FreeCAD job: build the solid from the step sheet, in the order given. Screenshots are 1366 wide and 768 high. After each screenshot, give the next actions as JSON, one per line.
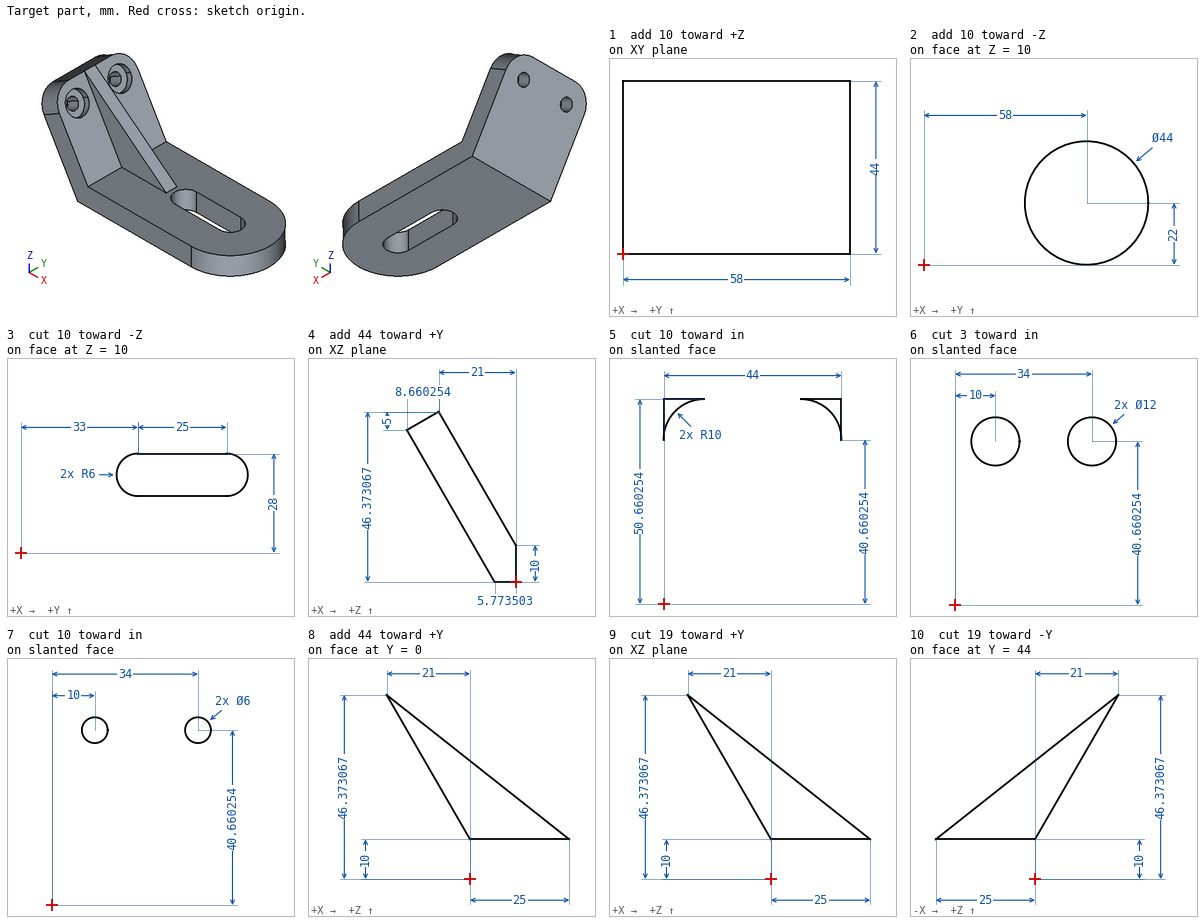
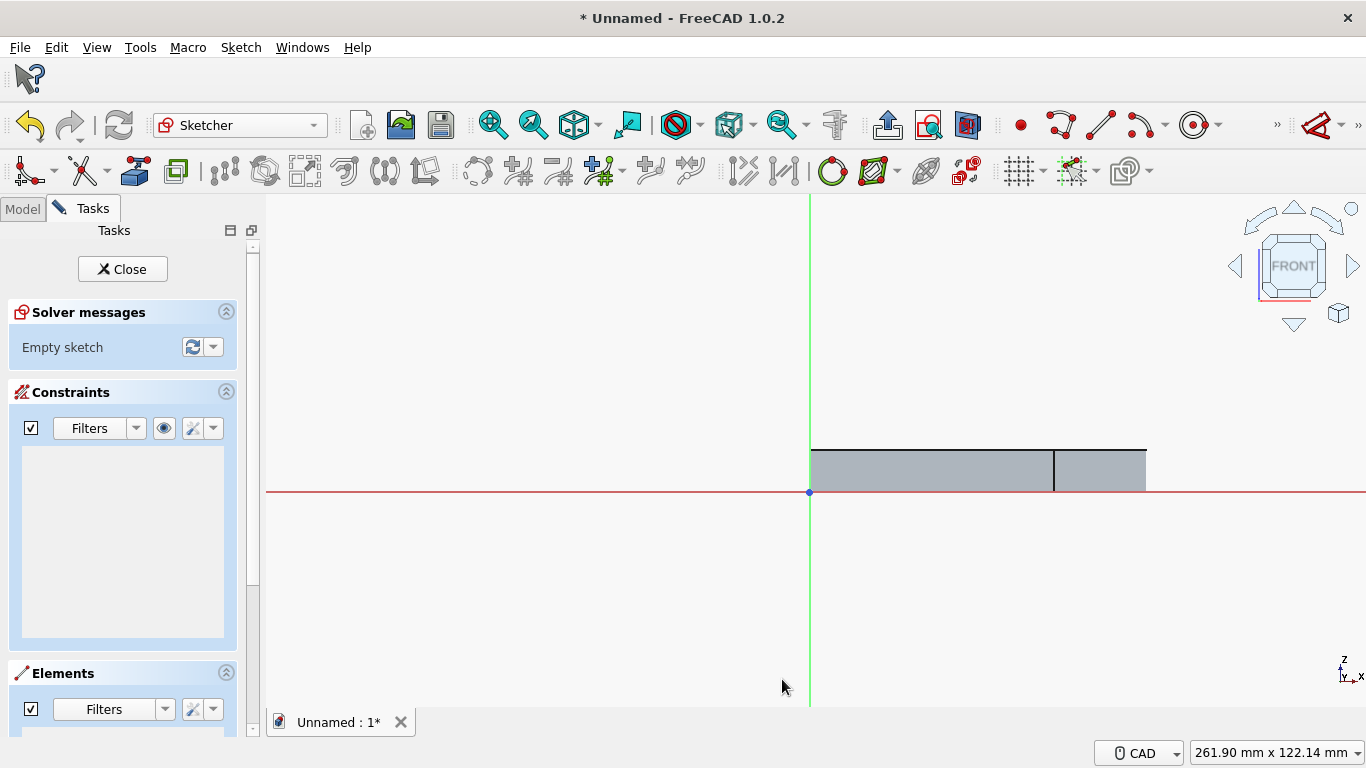
{"action": "scroll", "coordinate": [748, 327], "scroll_direction": "up", "scroll_amount": 3}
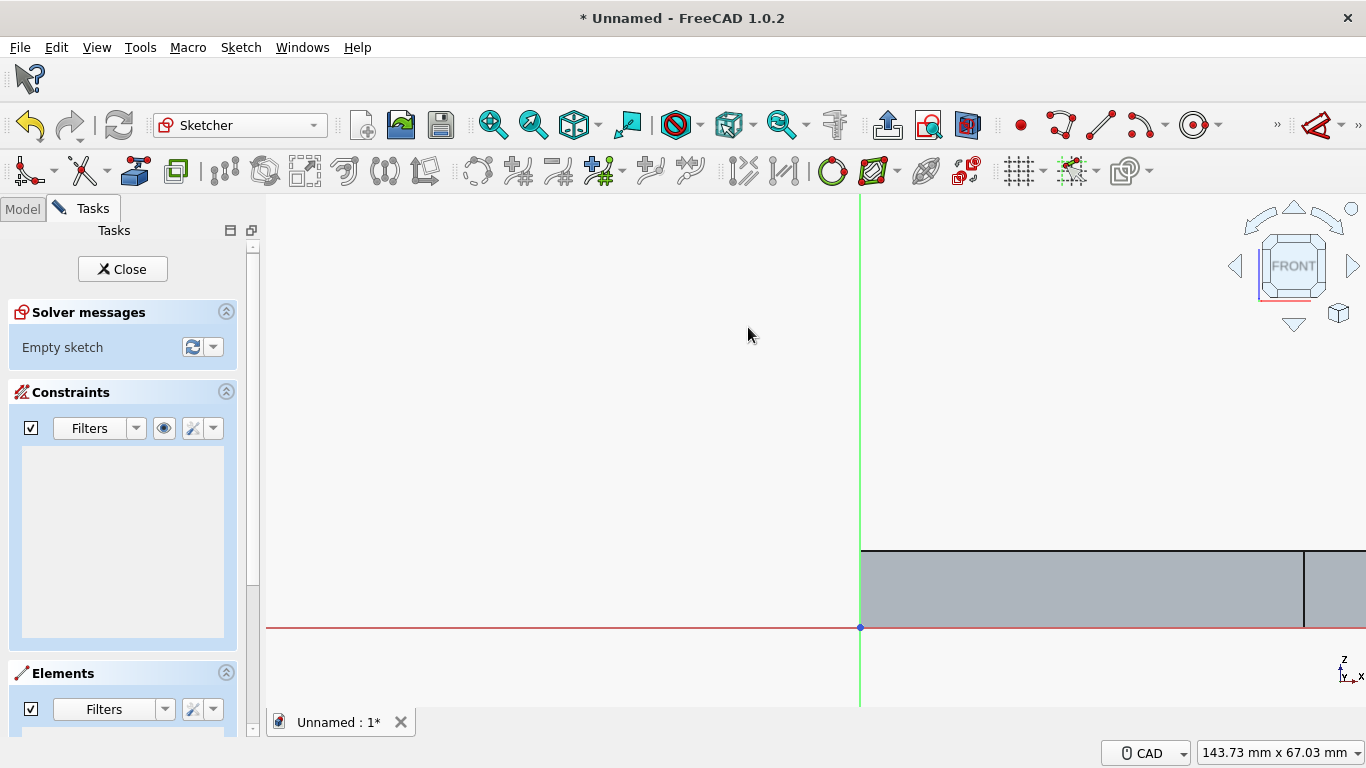
{"action": "left_click", "coordinate": [1062, 126]}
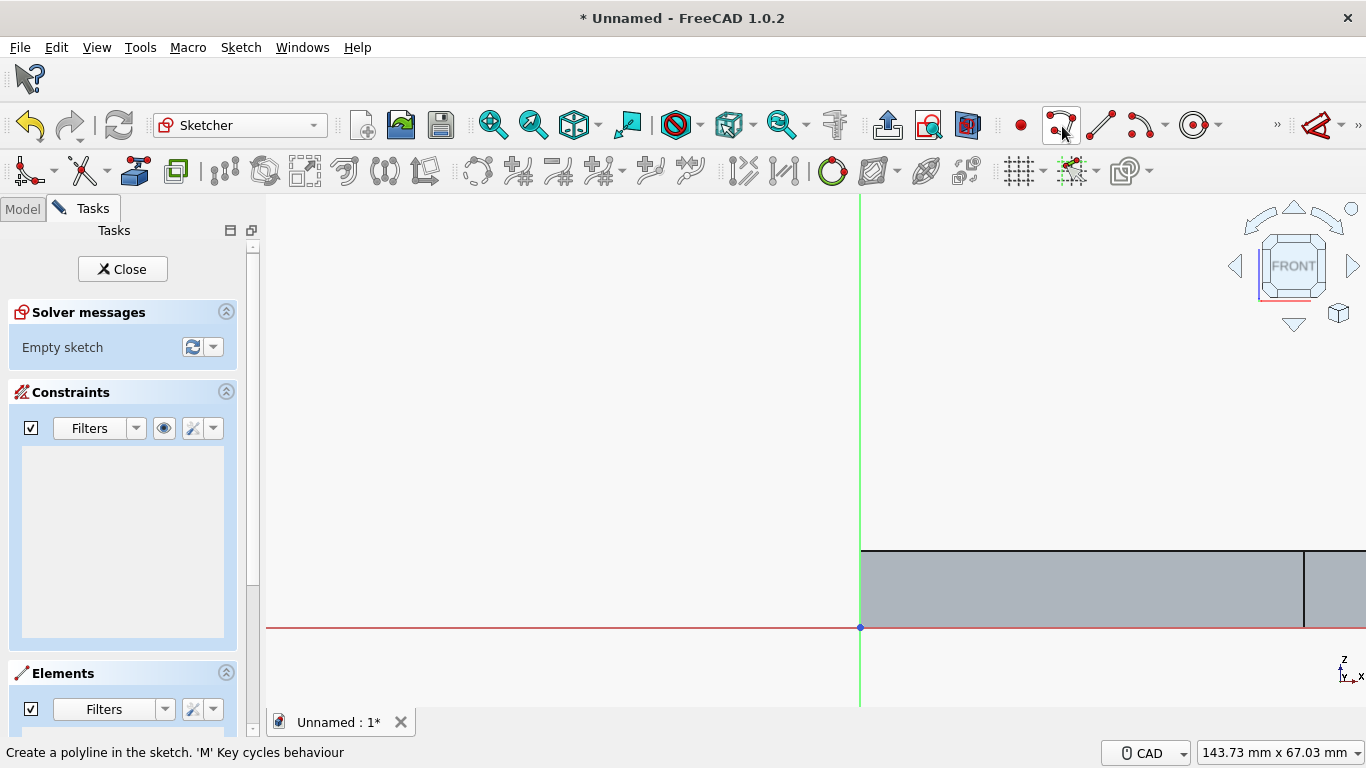
{"action": "left_click", "coordinate": [860, 628]}
{"action": "left_click", "coordinate": [851, 551]}
{"action": "left_click", "coordinate": [700, 273]}
{"action": "left_click", "coordinate": [633, 311]}
{"action": "left_click", "coordinate": [816, 619]}
{"action": "left_click", "coordinate": [860, 628]}
{"action": "key", "text": "Escape"}
{"action": "key", "text": "Escape"}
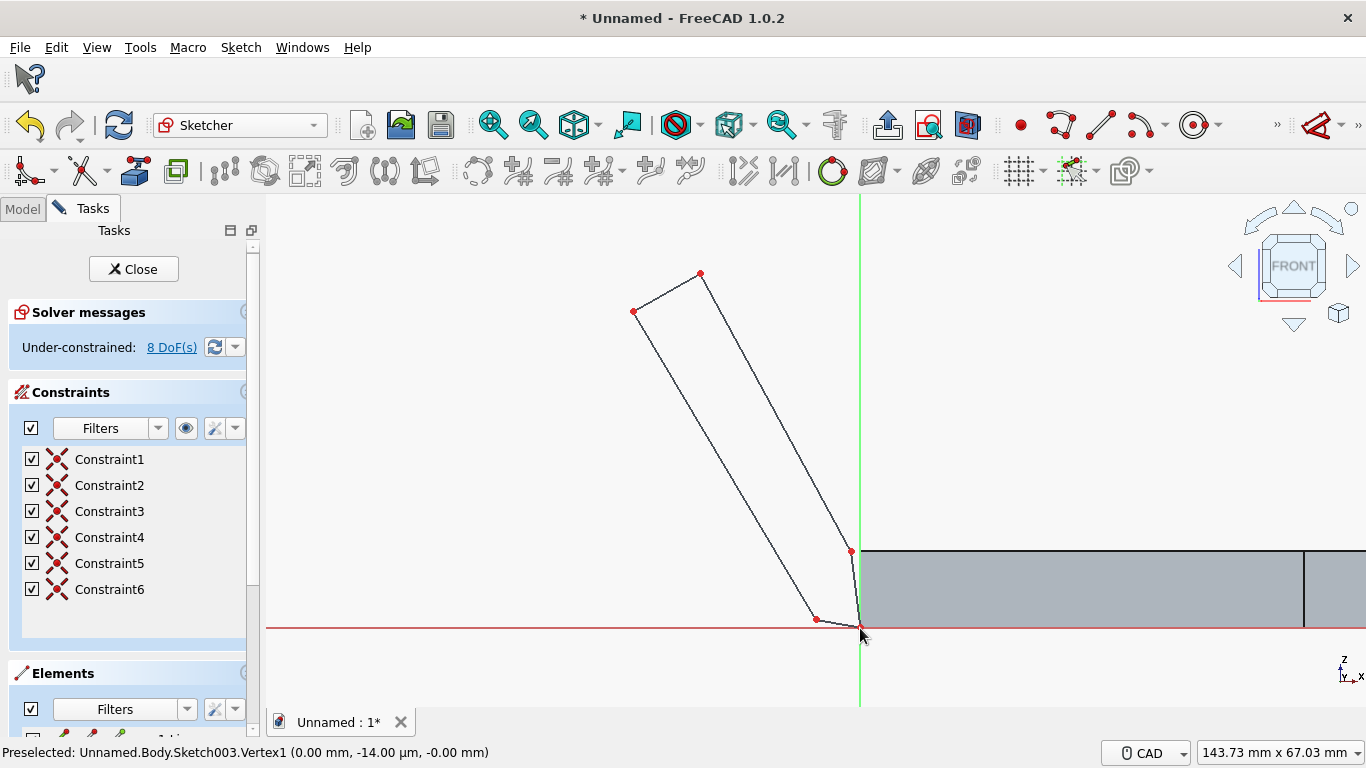
{"action": "left_click", "coordinate": [858, 605]}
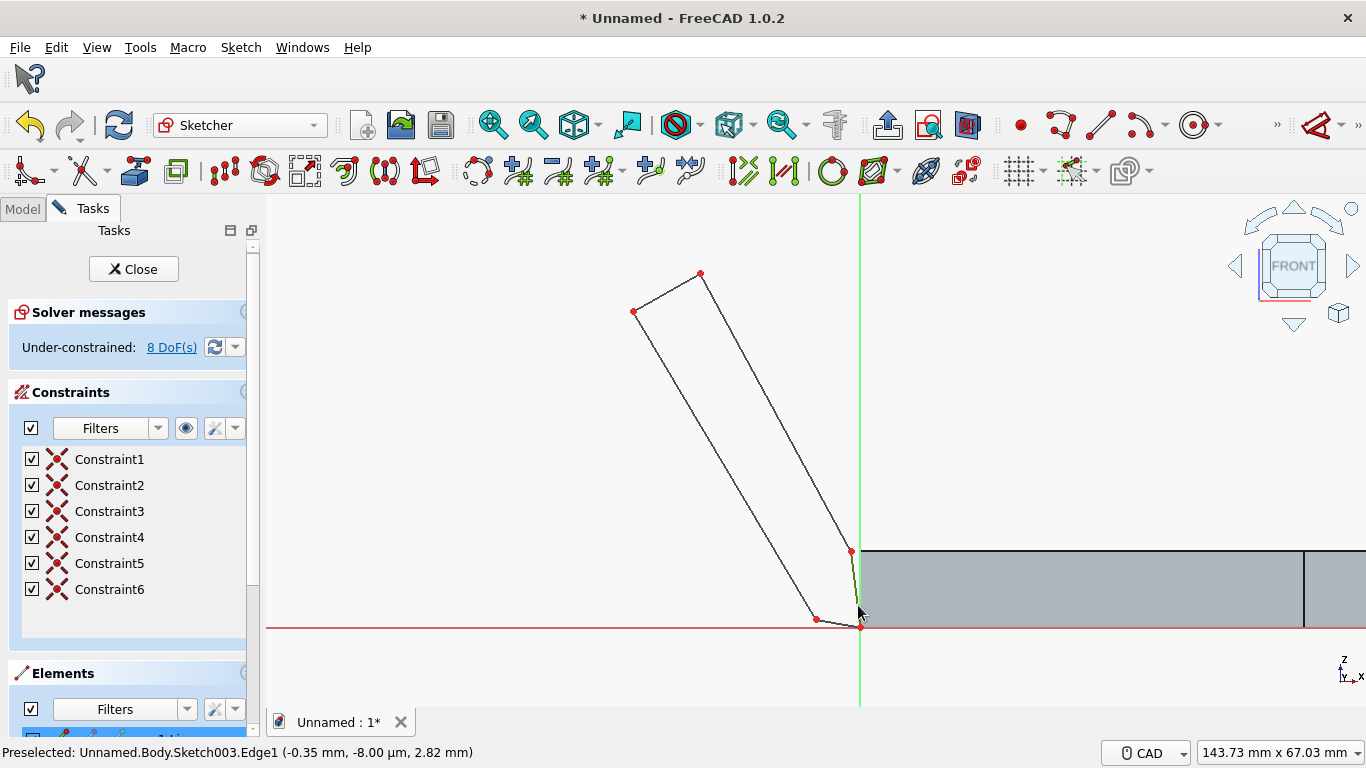
{"action": "key", "text": "v"}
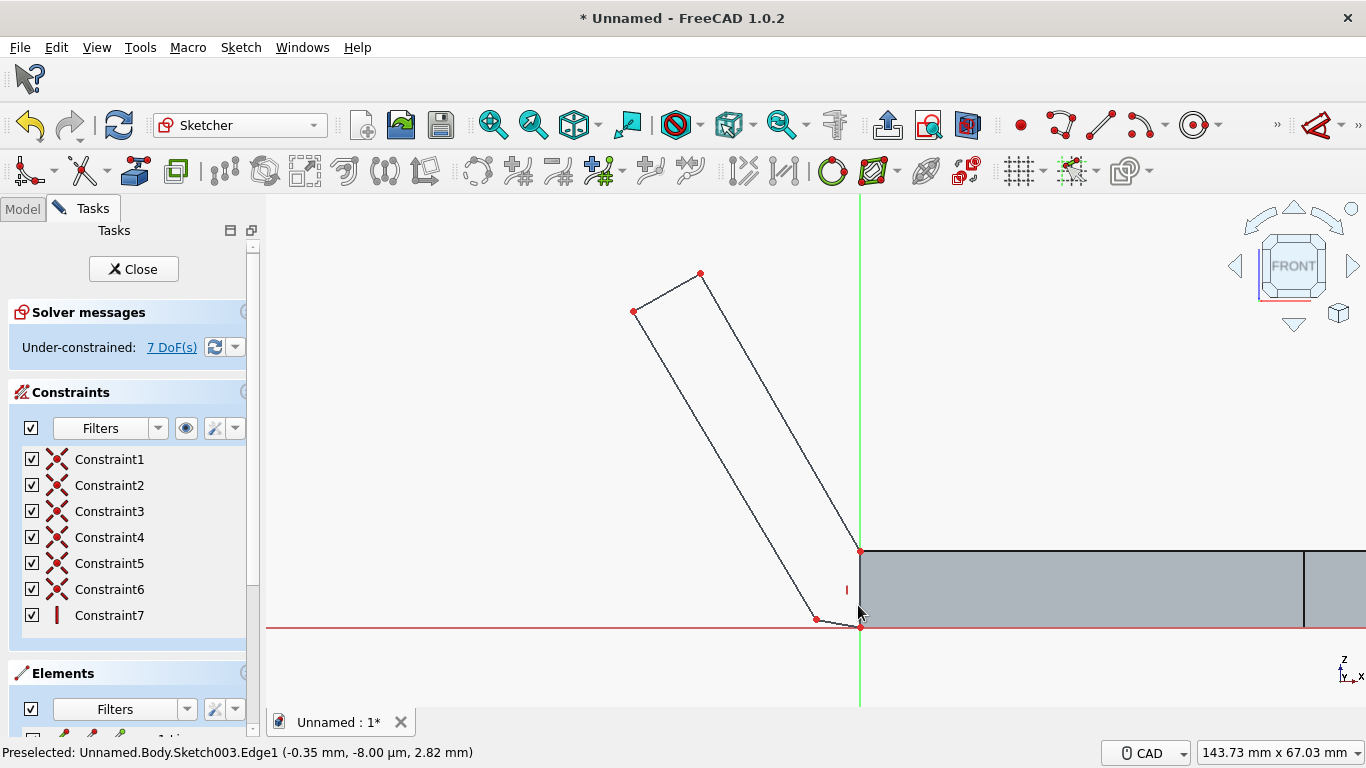
{"action": "left_click", "coordinate": [847, 625]}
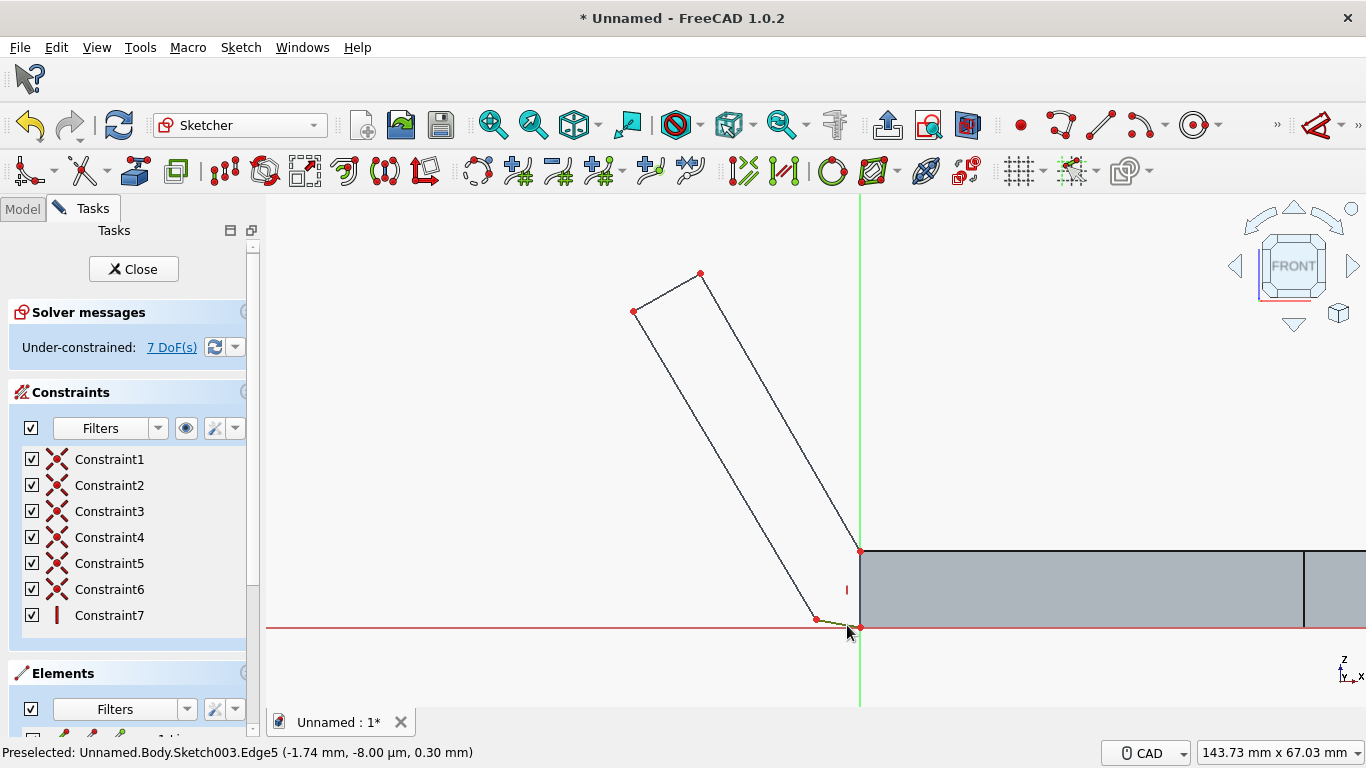
{"action": "key", "text": "h"}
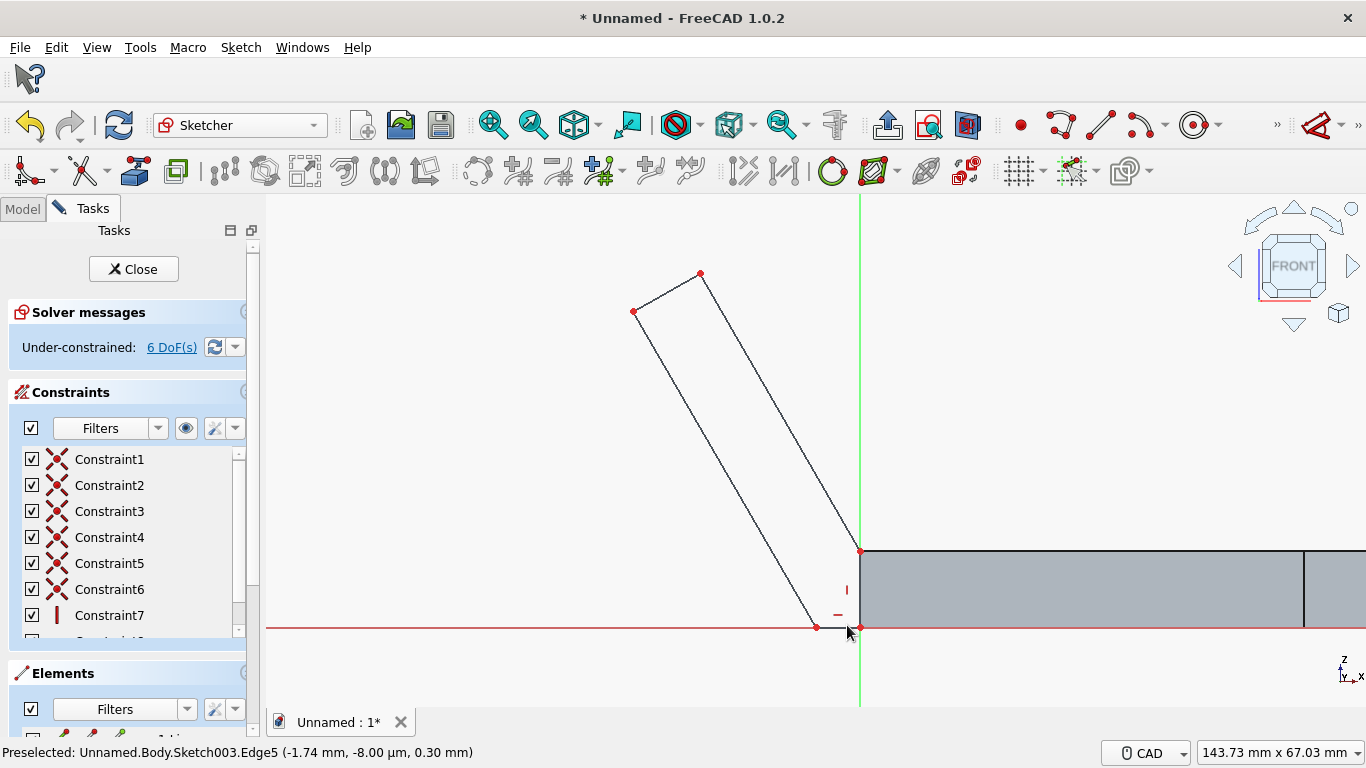
{"action": "key", "text": "d"}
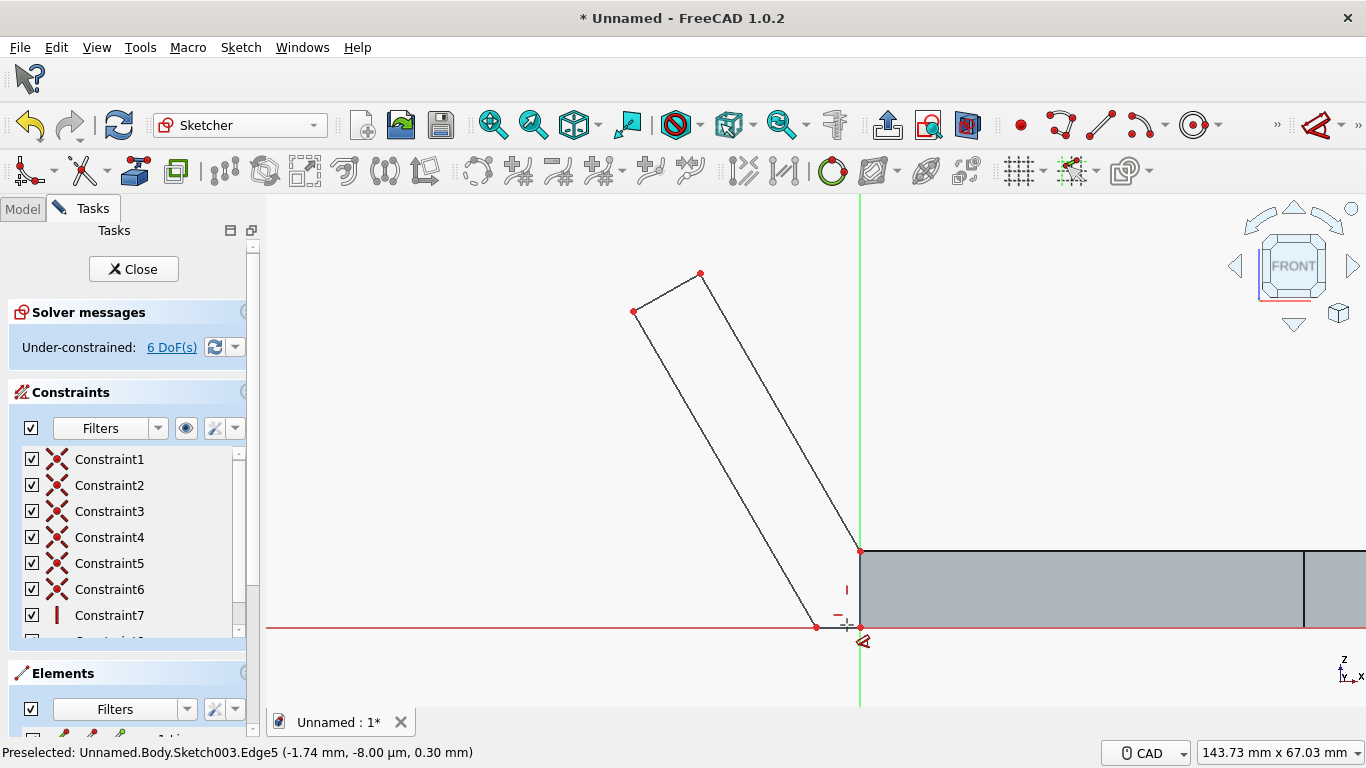
{"action": "left_click", "coordinate": [860, 605]}
{"action": "left_click", "coordinate": [894, 590]}